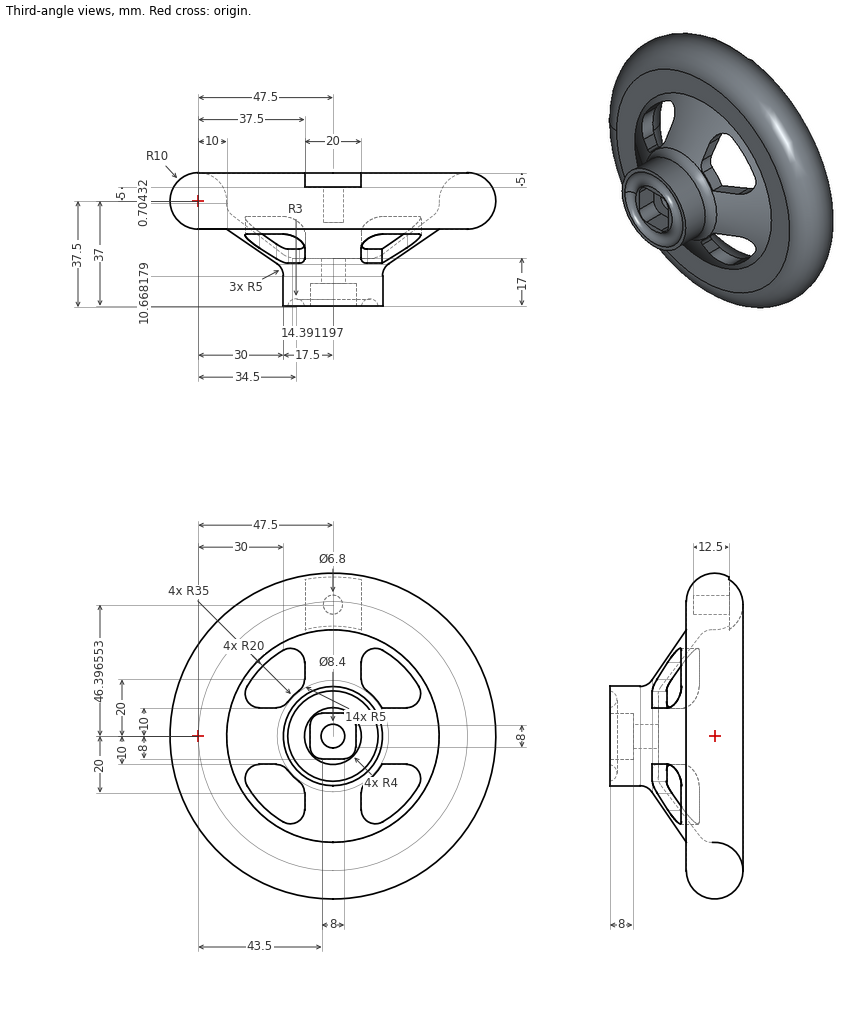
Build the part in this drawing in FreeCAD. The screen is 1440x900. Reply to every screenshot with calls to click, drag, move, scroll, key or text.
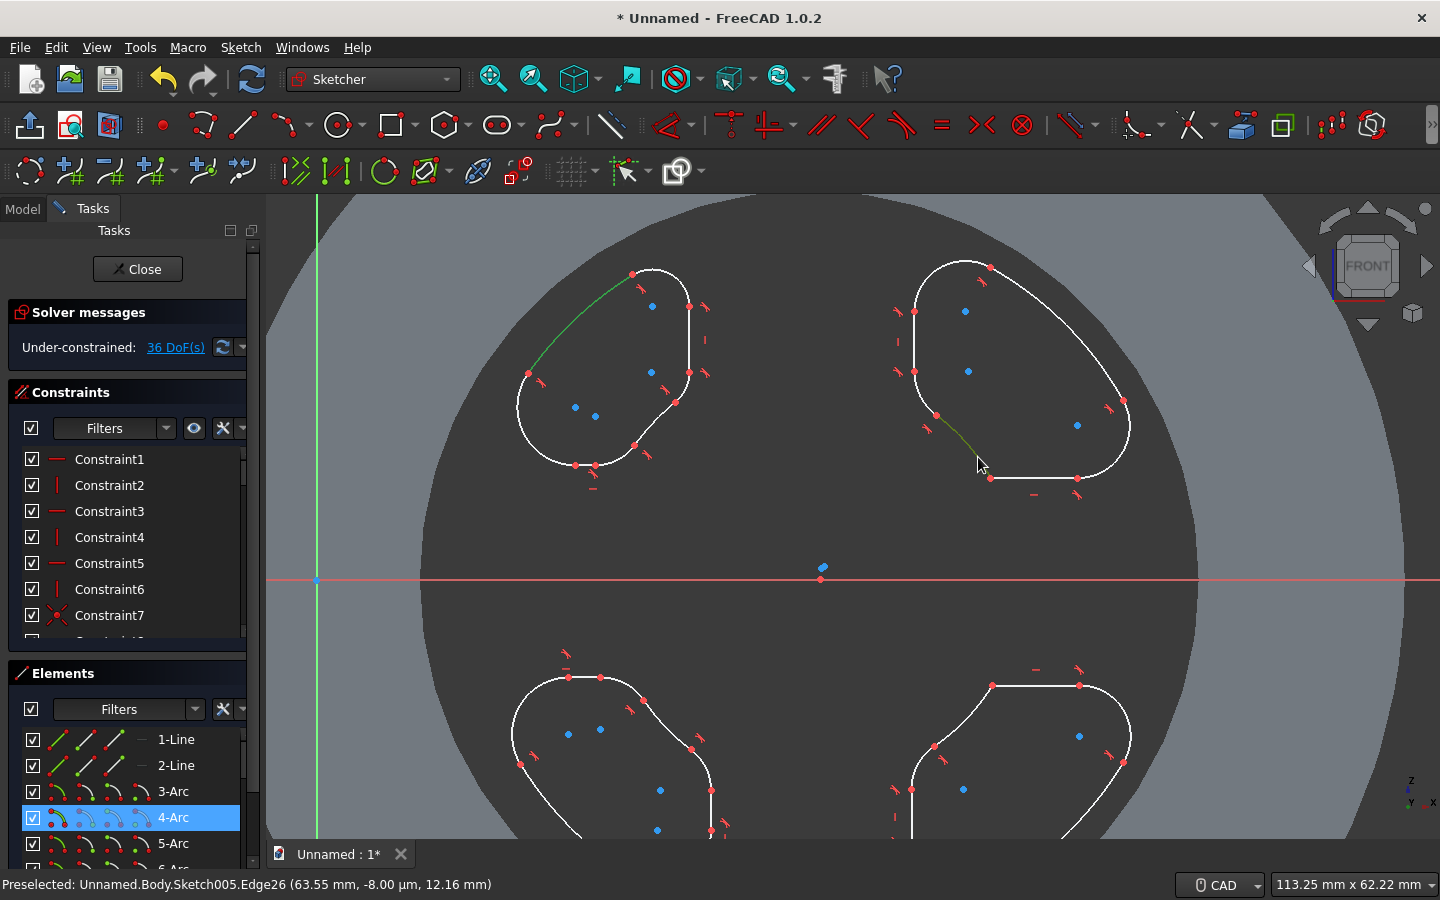
click(730, 126)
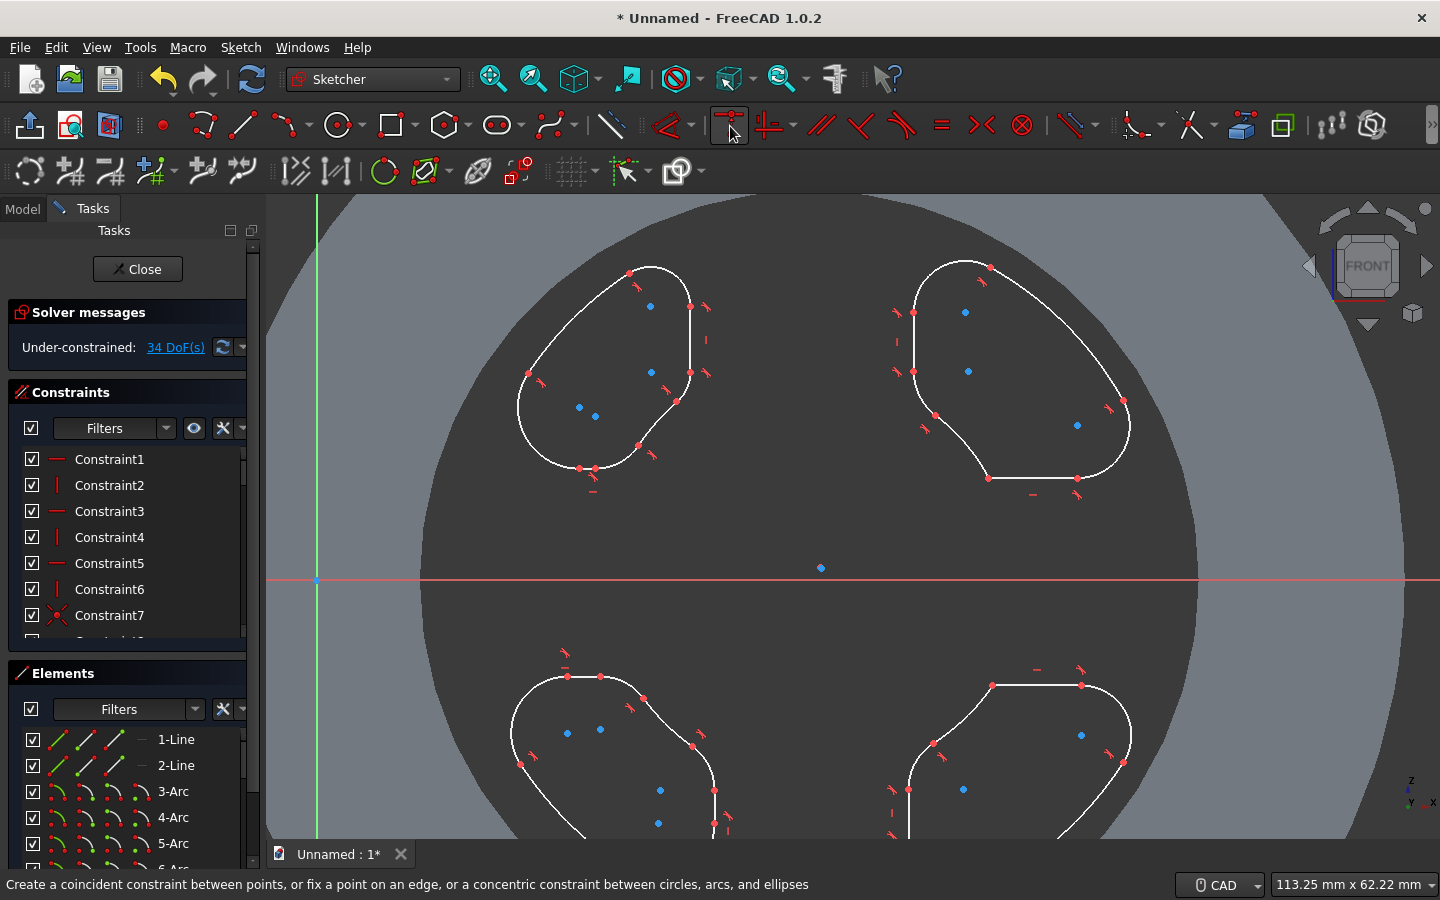
click(595, 299)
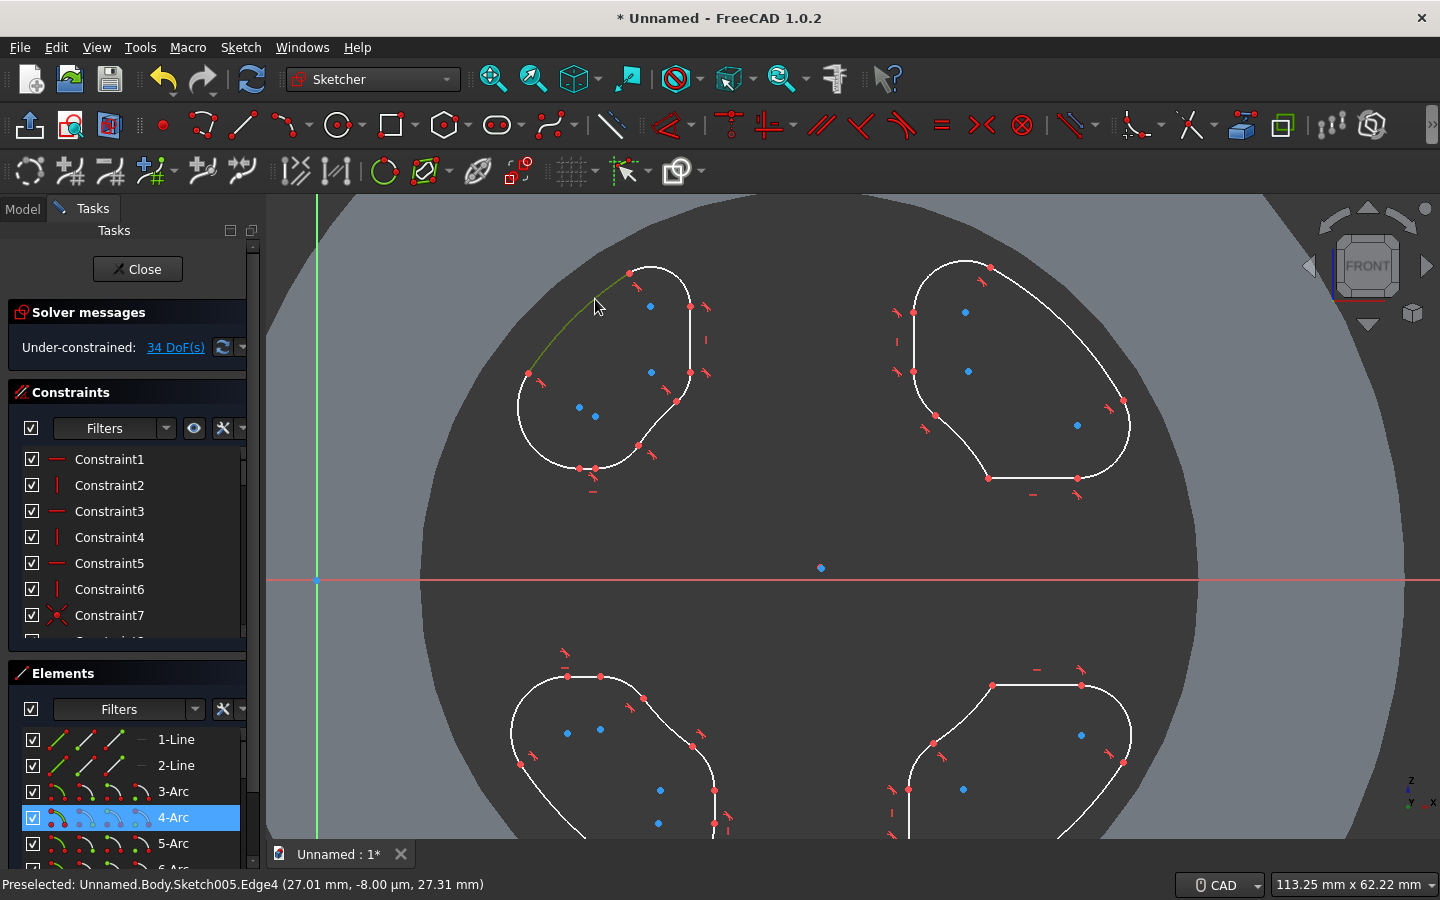
click(1091, 353)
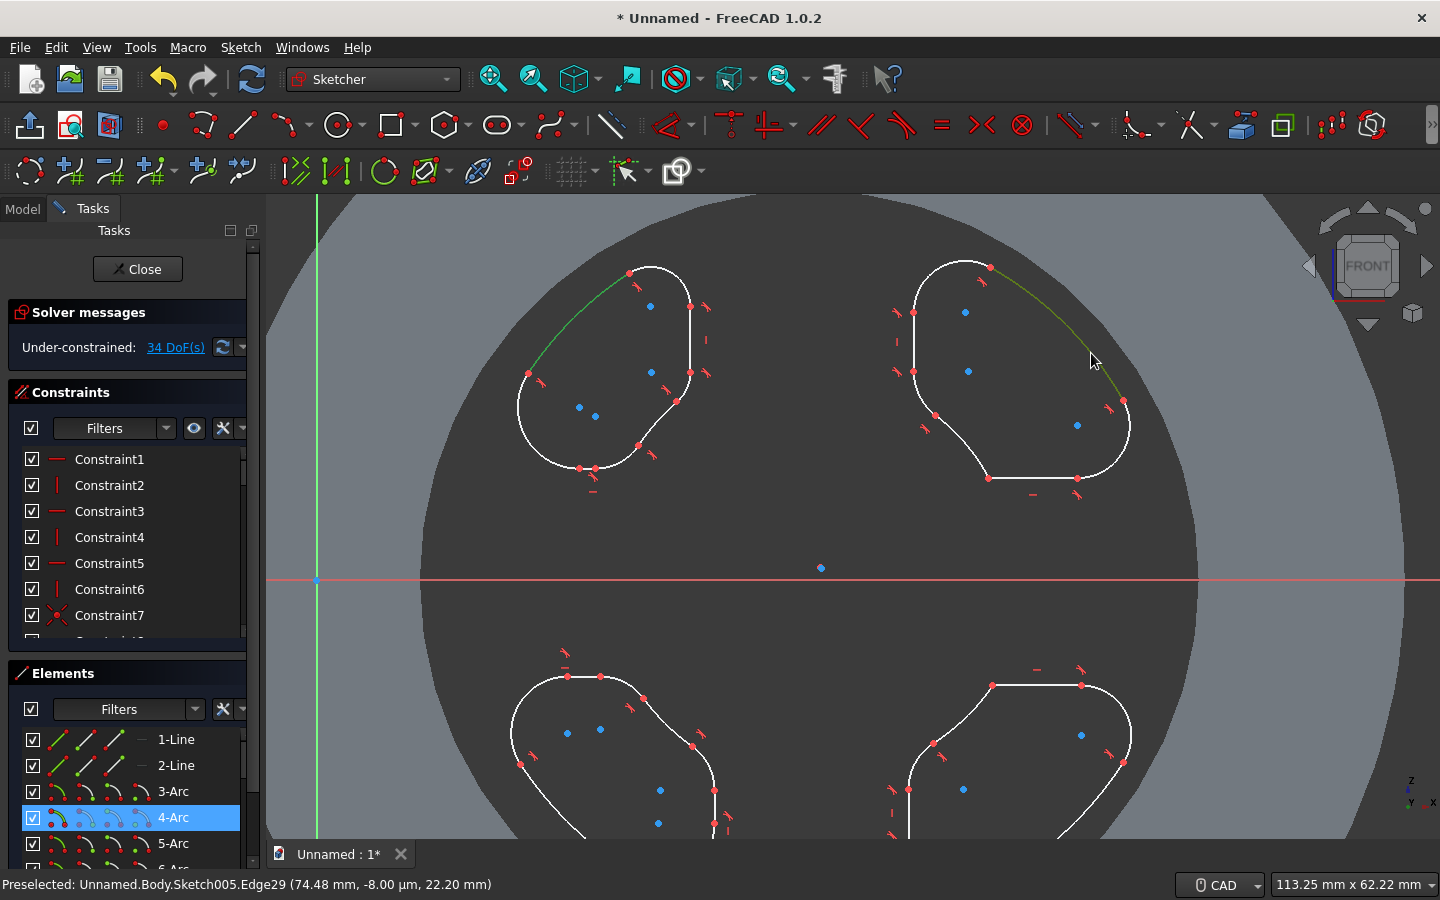
click(730, 126)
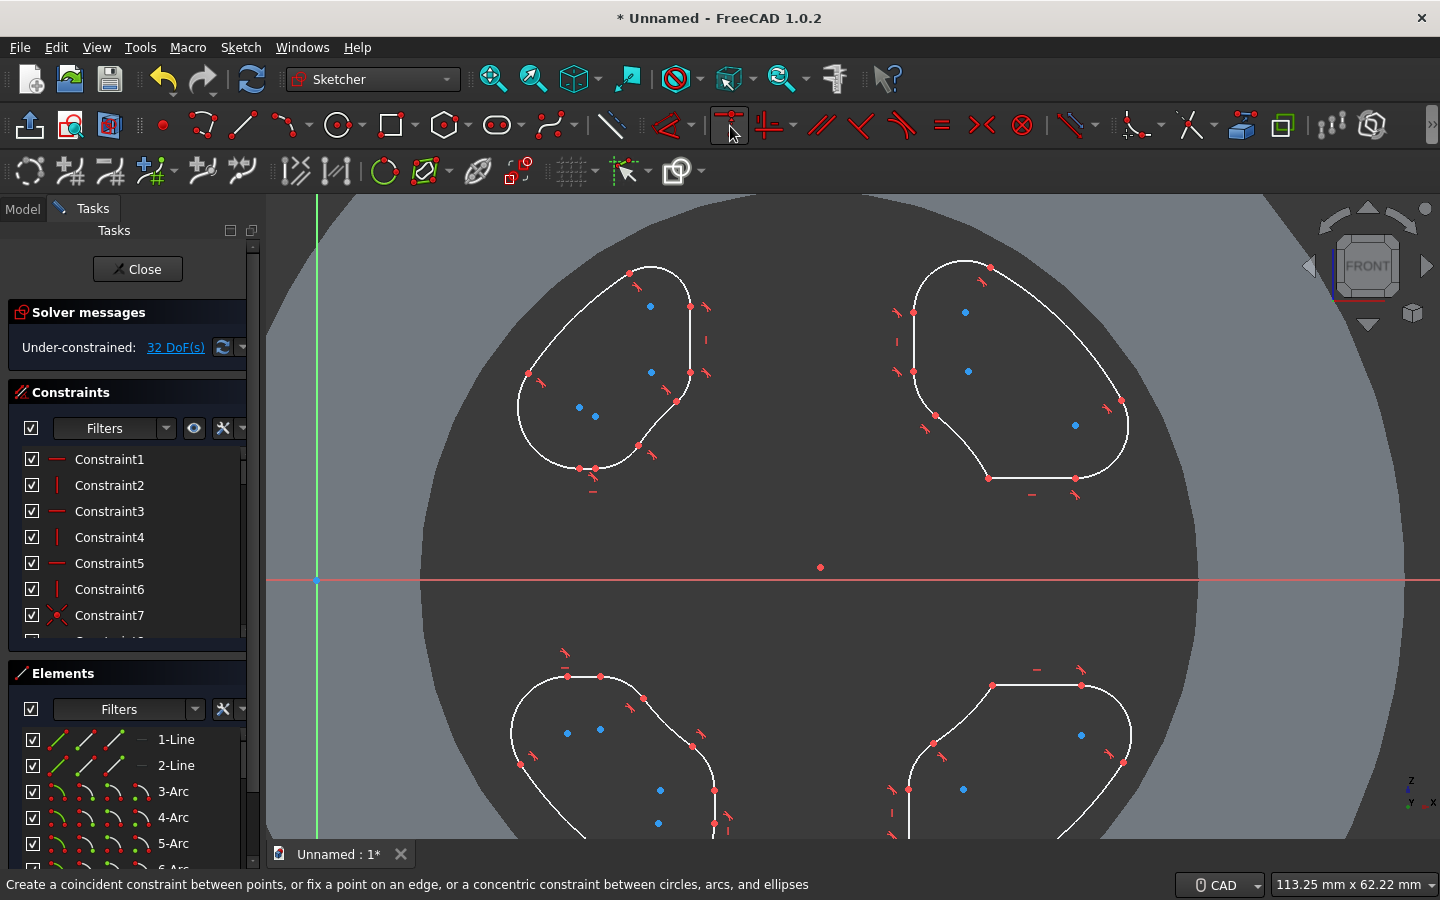
click(518, 411)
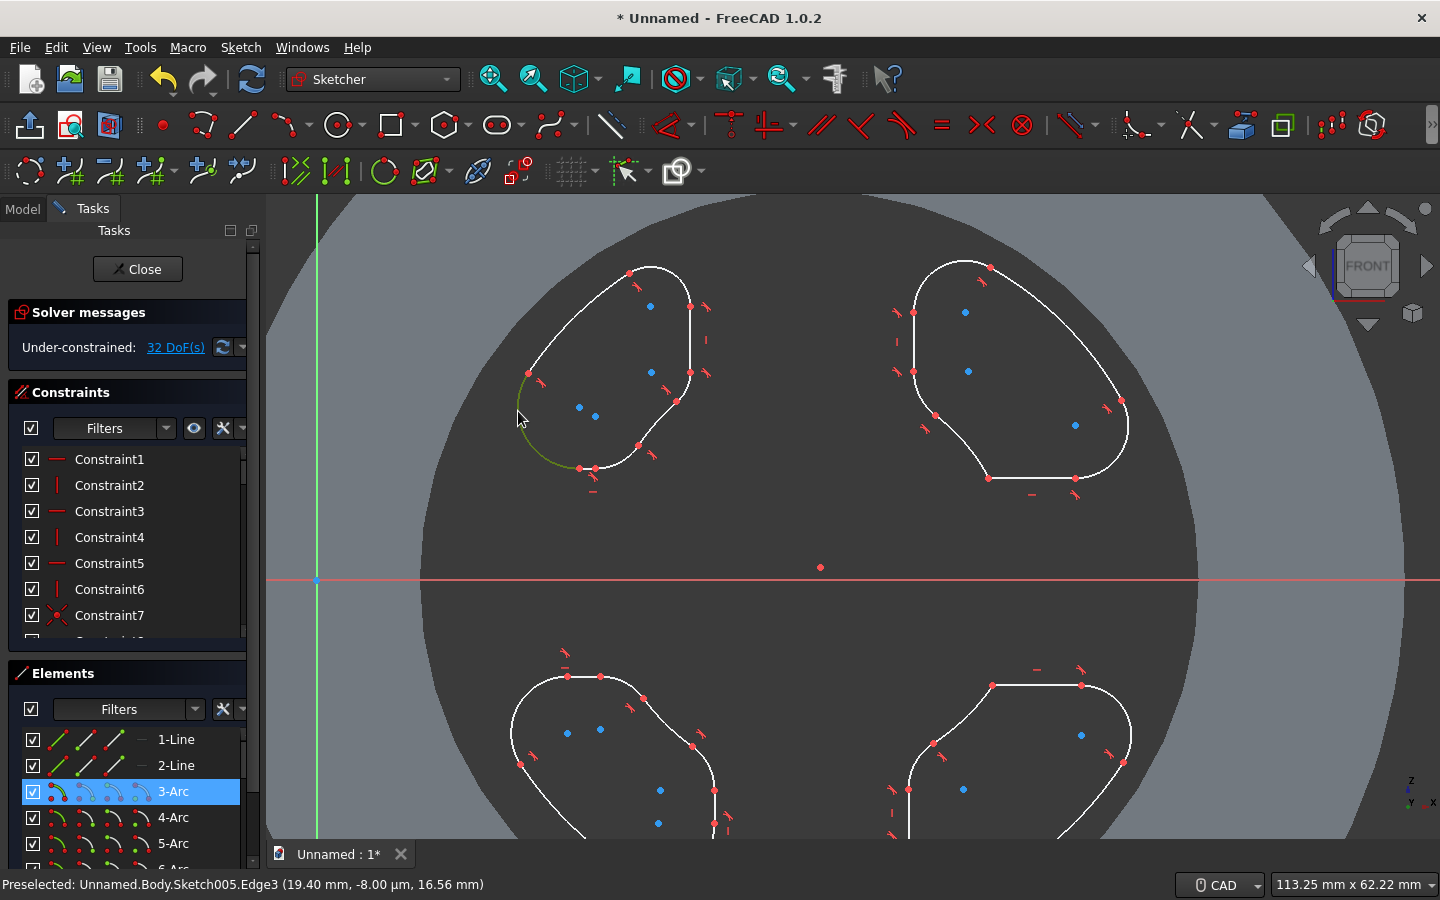
click(682, 283)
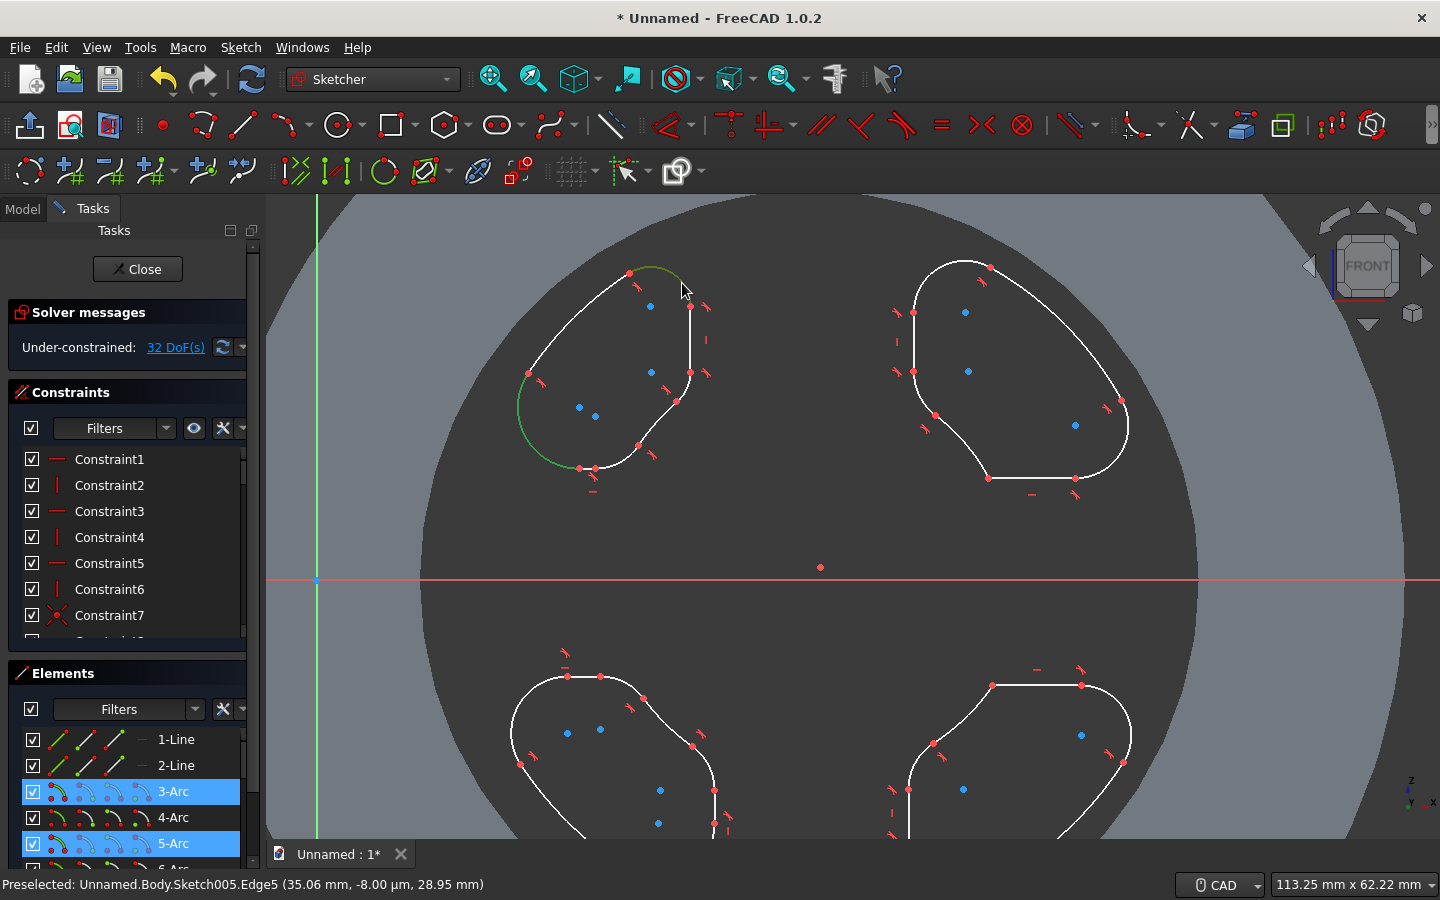
scroll(684, 395, up, 2)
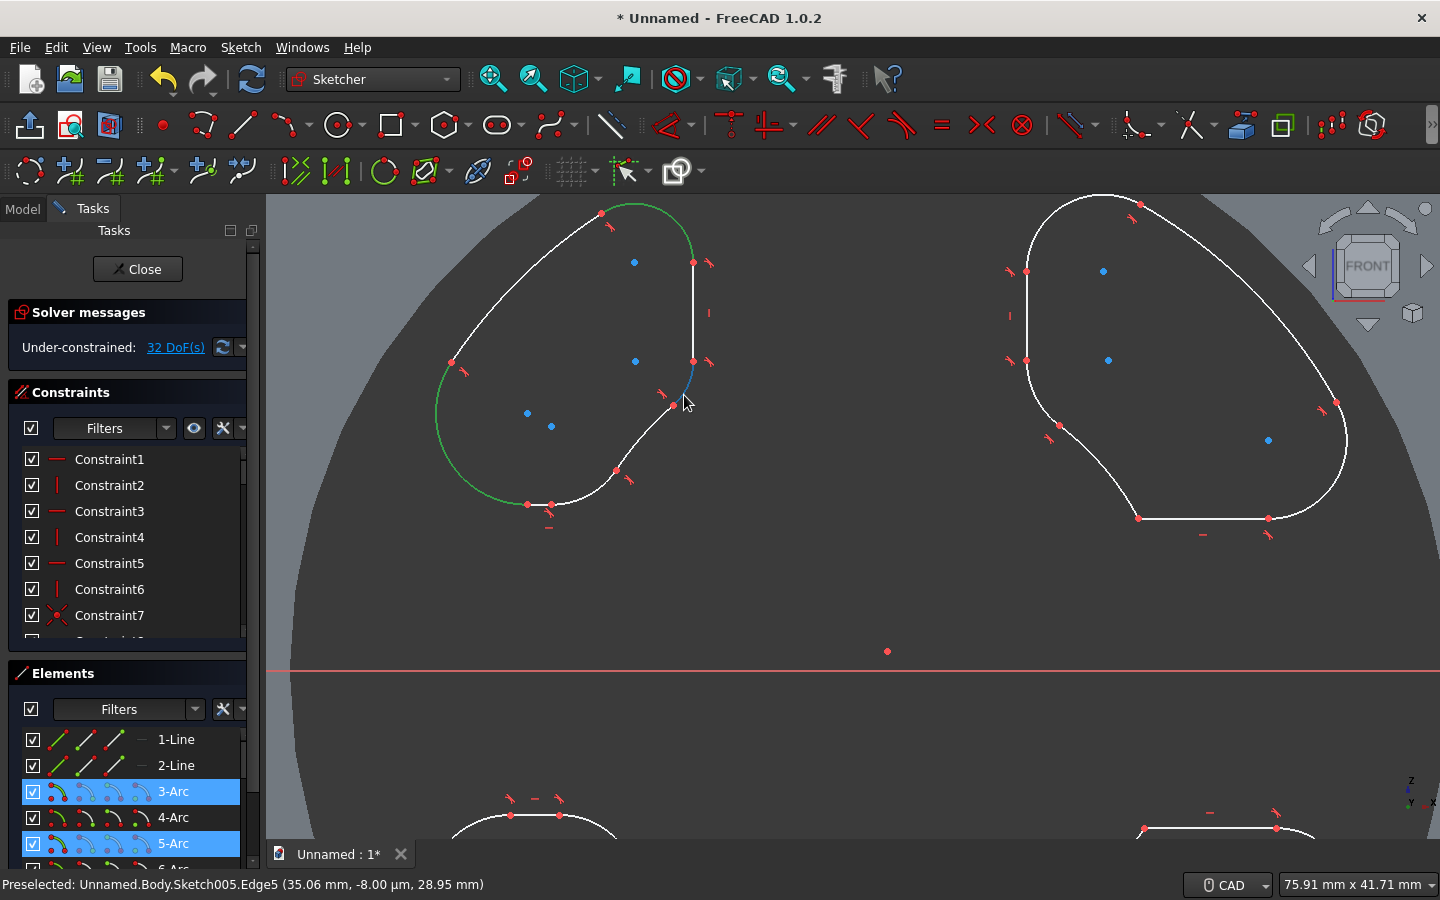
click(683, 394)